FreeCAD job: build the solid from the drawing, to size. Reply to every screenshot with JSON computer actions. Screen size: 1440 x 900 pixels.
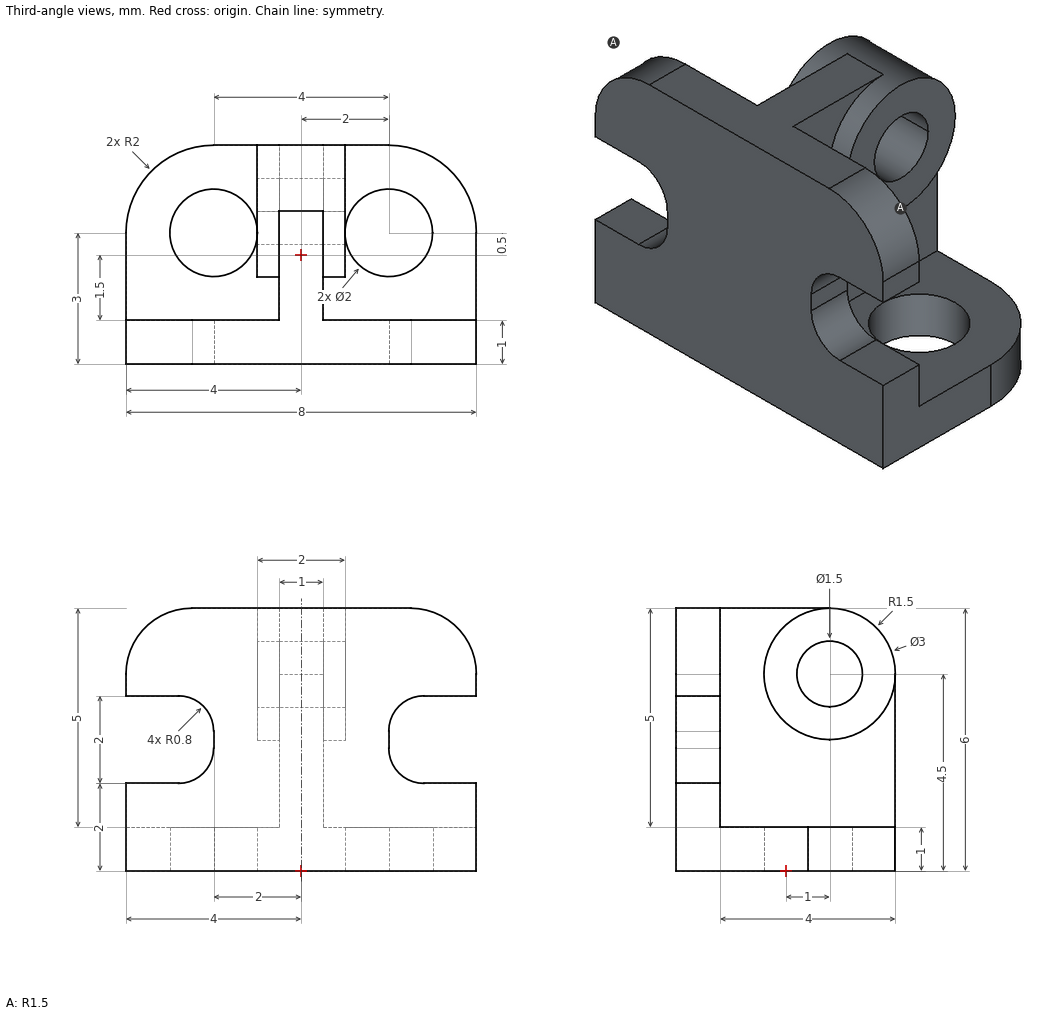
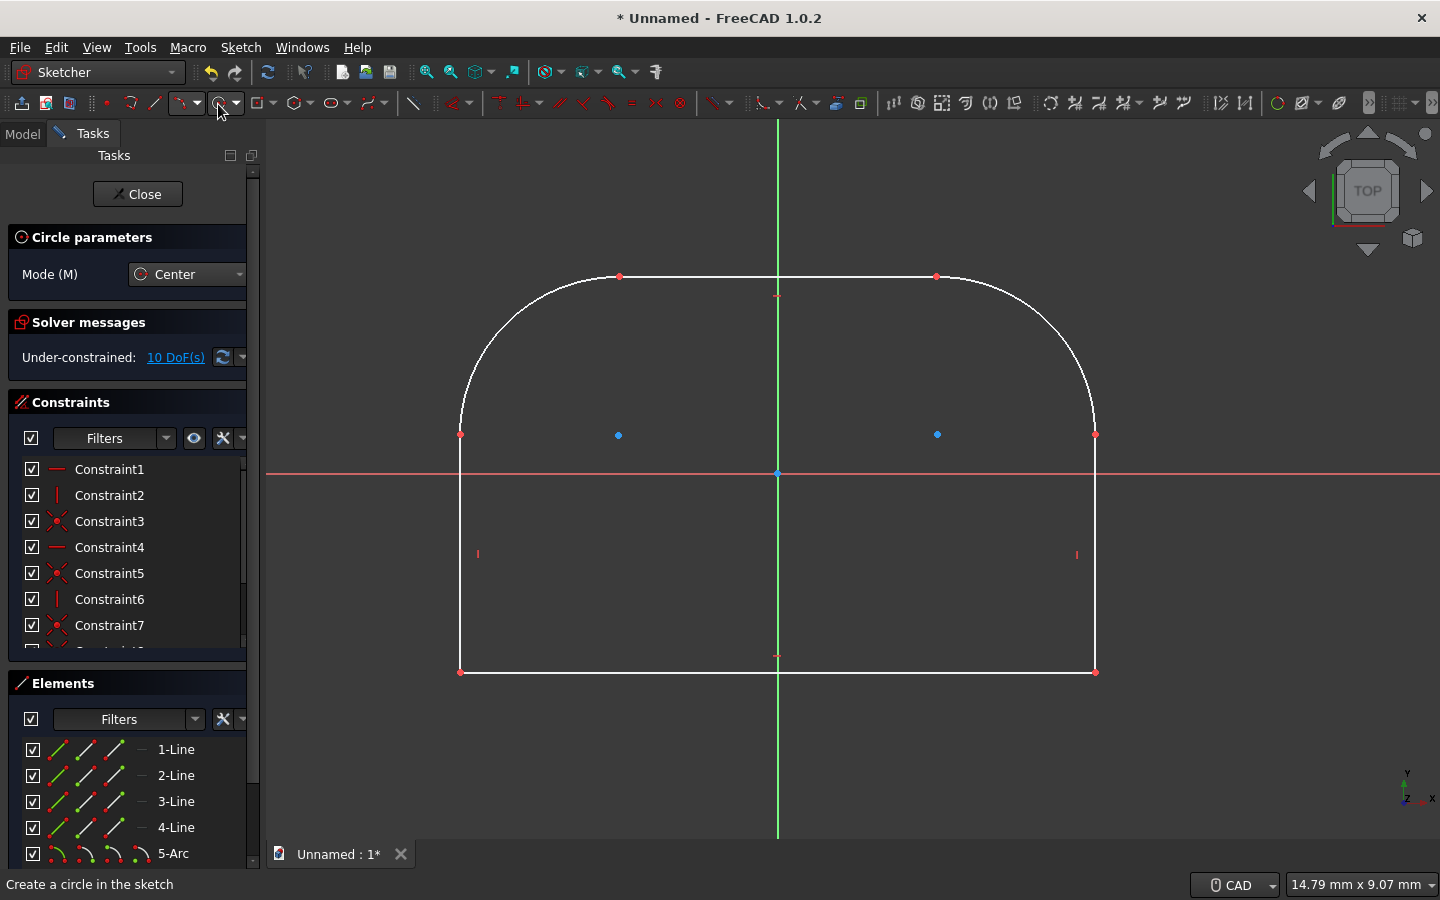
{"action": "left_click", "coordinate": [936, 434]}
{"action": "mouse_move", "coordinate": [993, 378]}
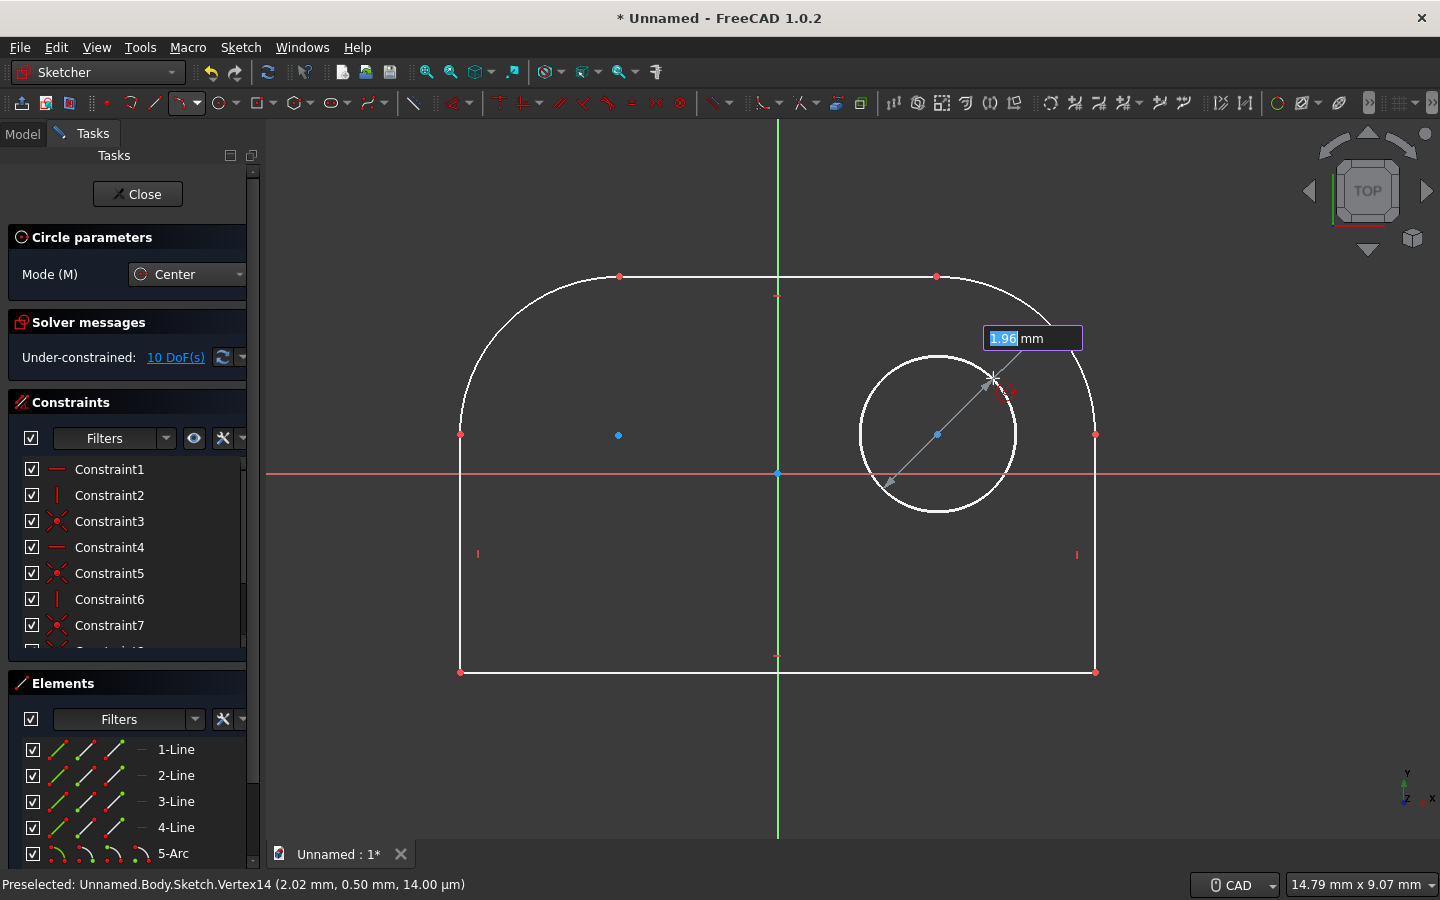
{"action": "type", "text": "2"}
{"action": "key", "text": "Return"}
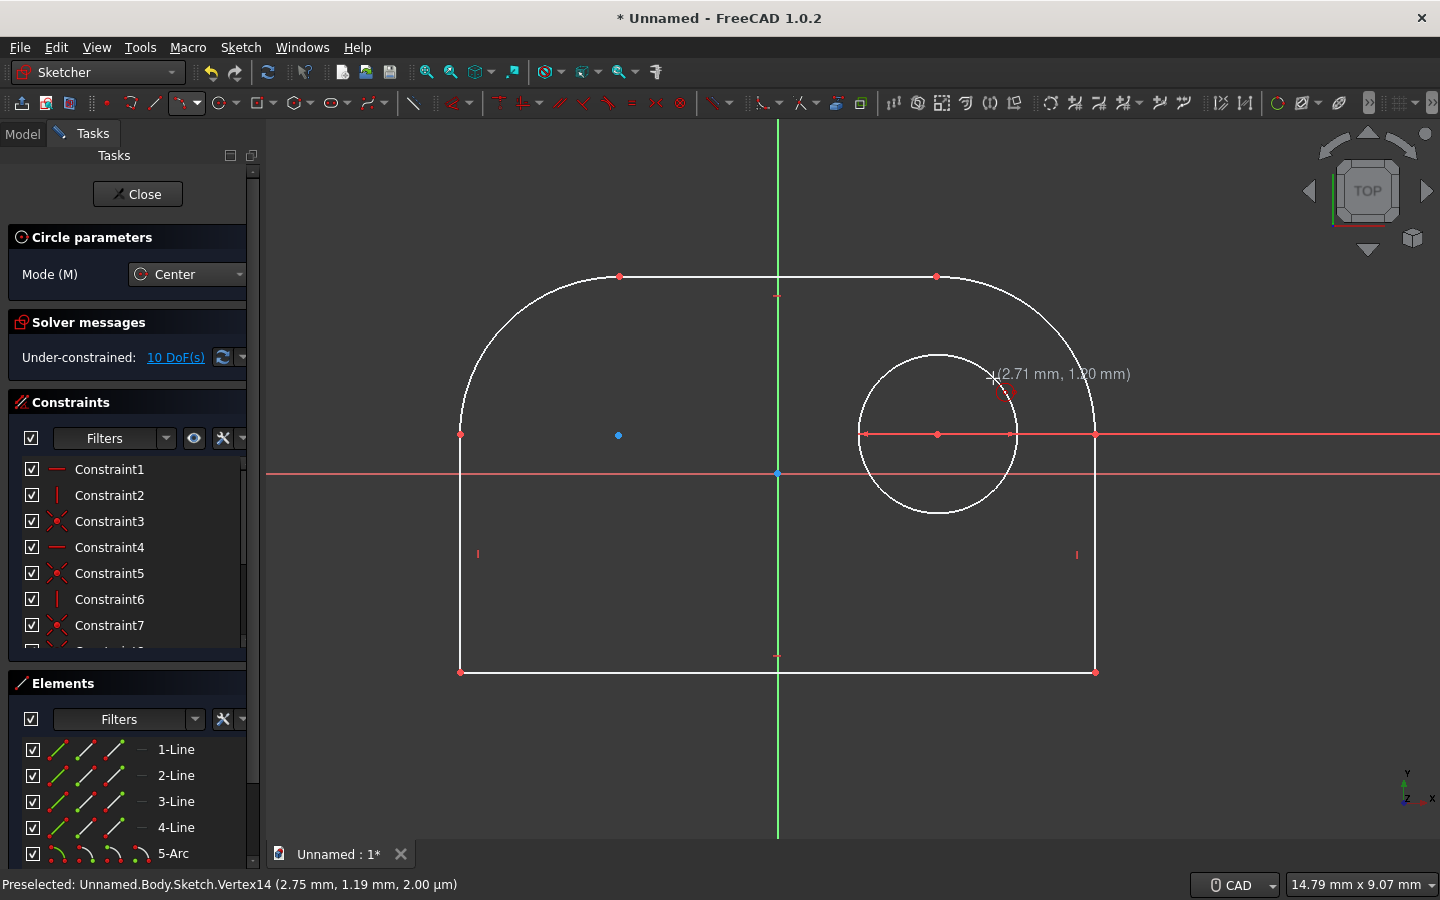
{"action": "left_click", "coordinate": [619, 434]}
{"action": "mouse_move", "coordinate": [675, 378]}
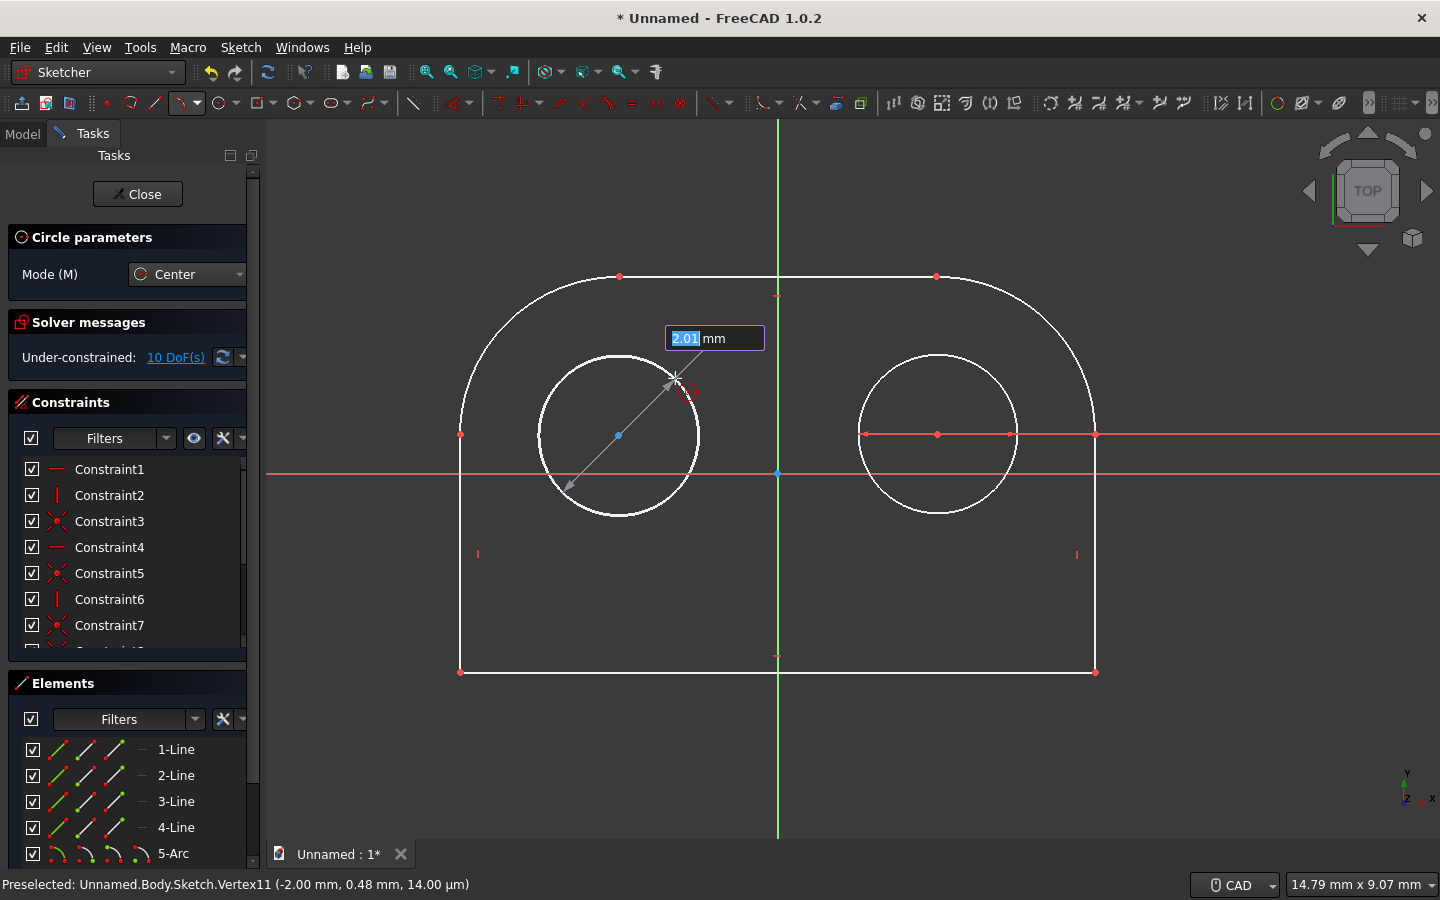
{"action": "type", "text": "2"}
{"action": "key", "text": "Return"}
{"action": "key", "text": "Escape"}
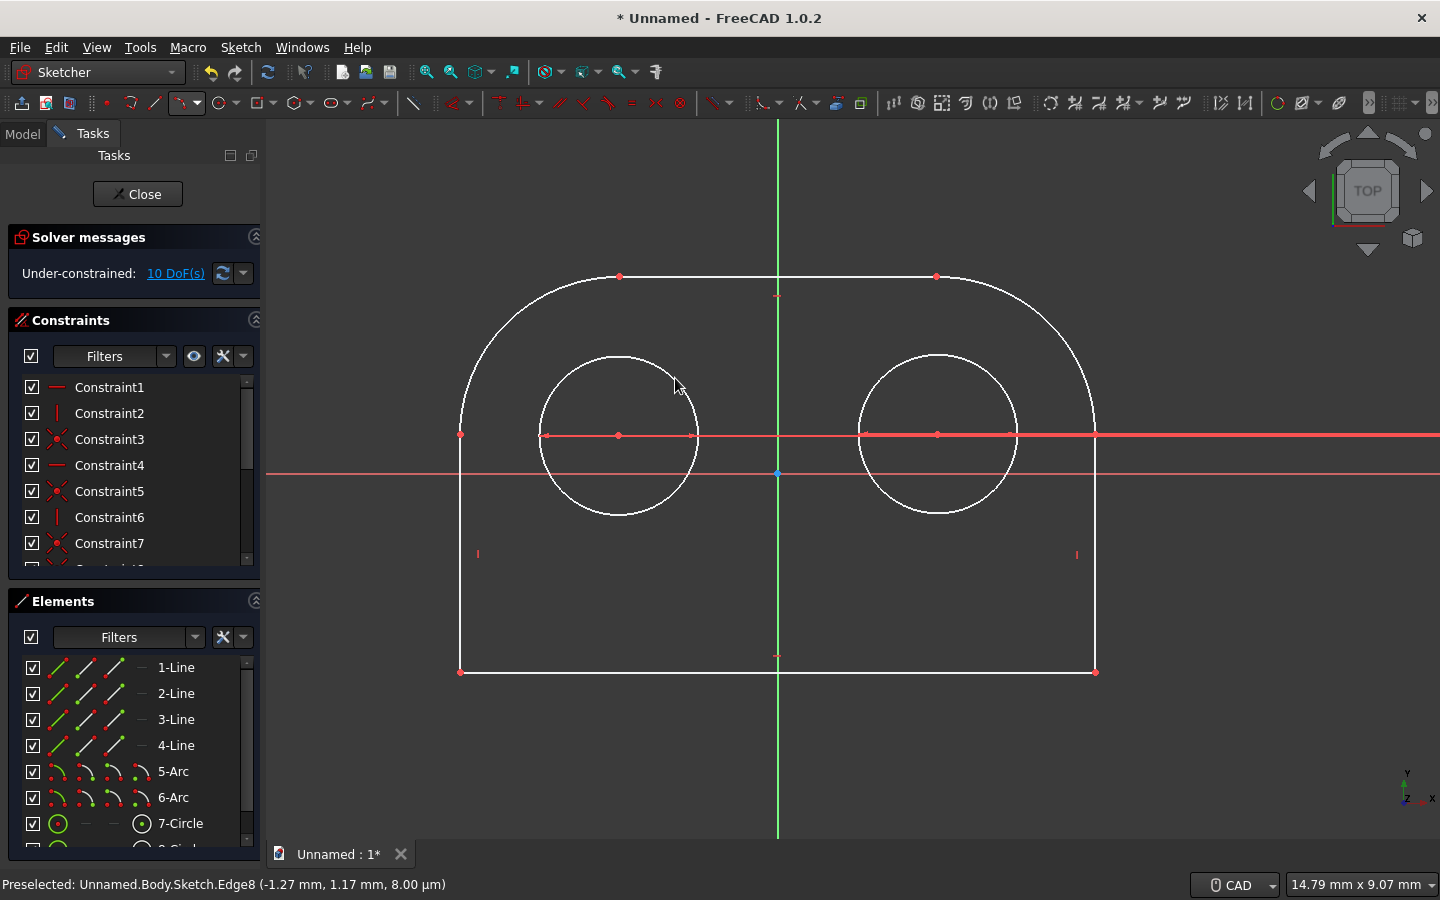
{"action": "left_click", "coordinate": [841, 277]}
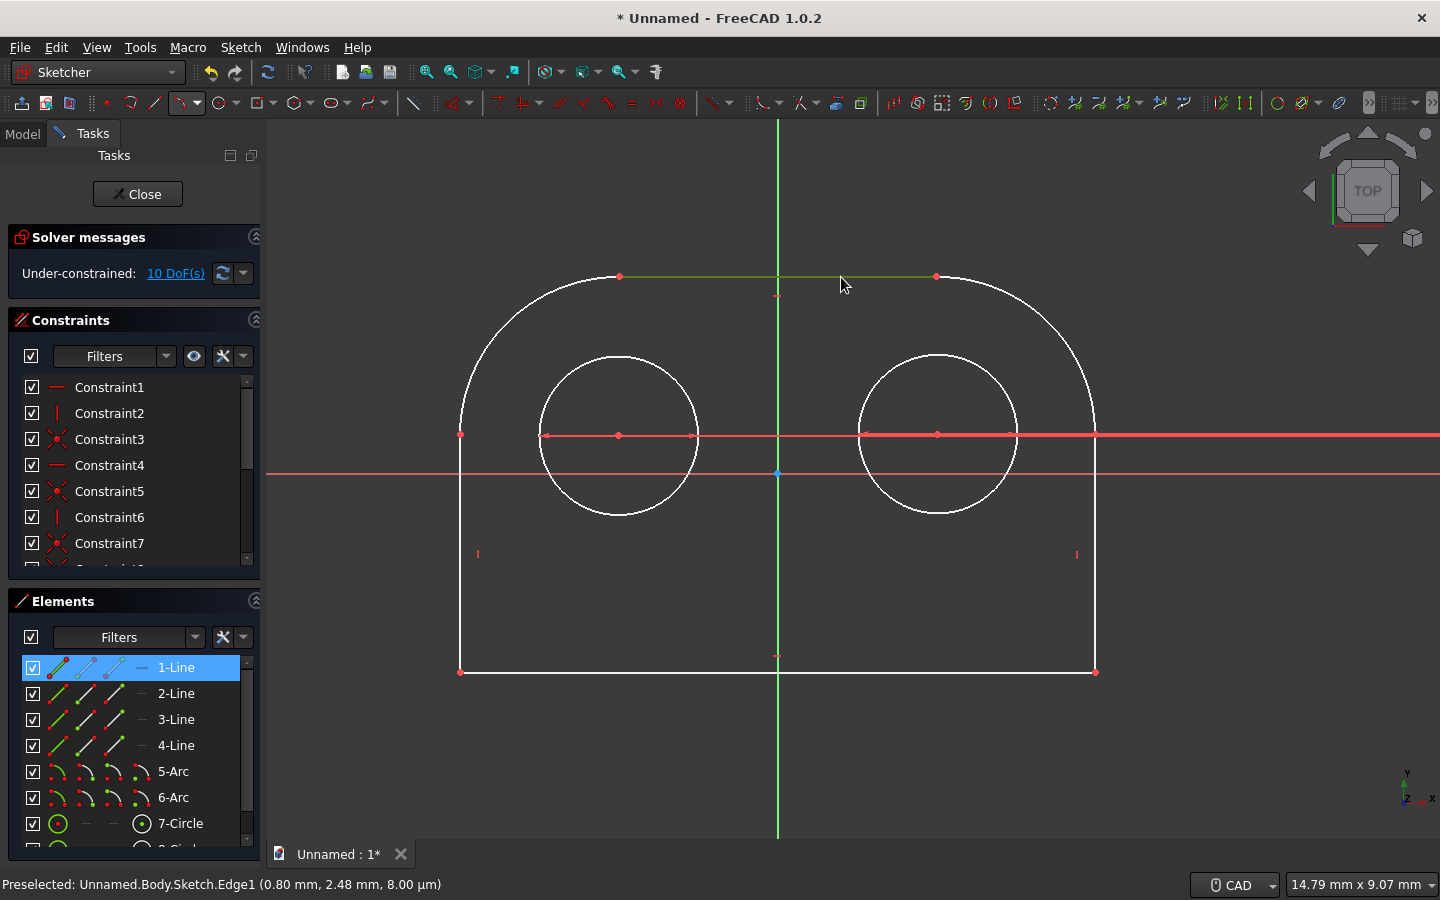
{"action": "left_click", "coordinate": [547, 294]}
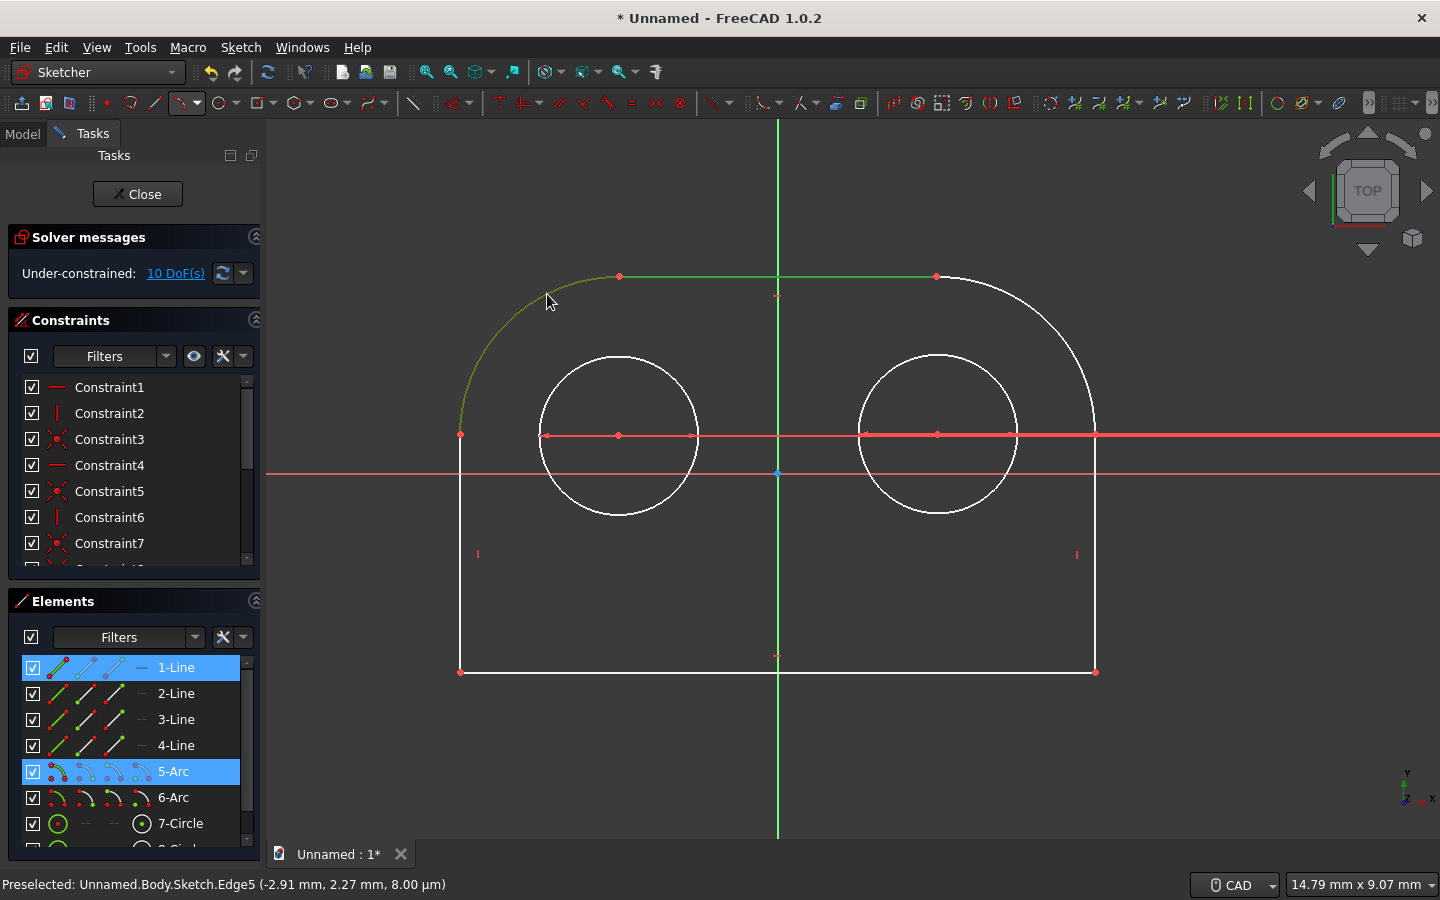
{"action": "left_click", "coordinate": [608, 104]}